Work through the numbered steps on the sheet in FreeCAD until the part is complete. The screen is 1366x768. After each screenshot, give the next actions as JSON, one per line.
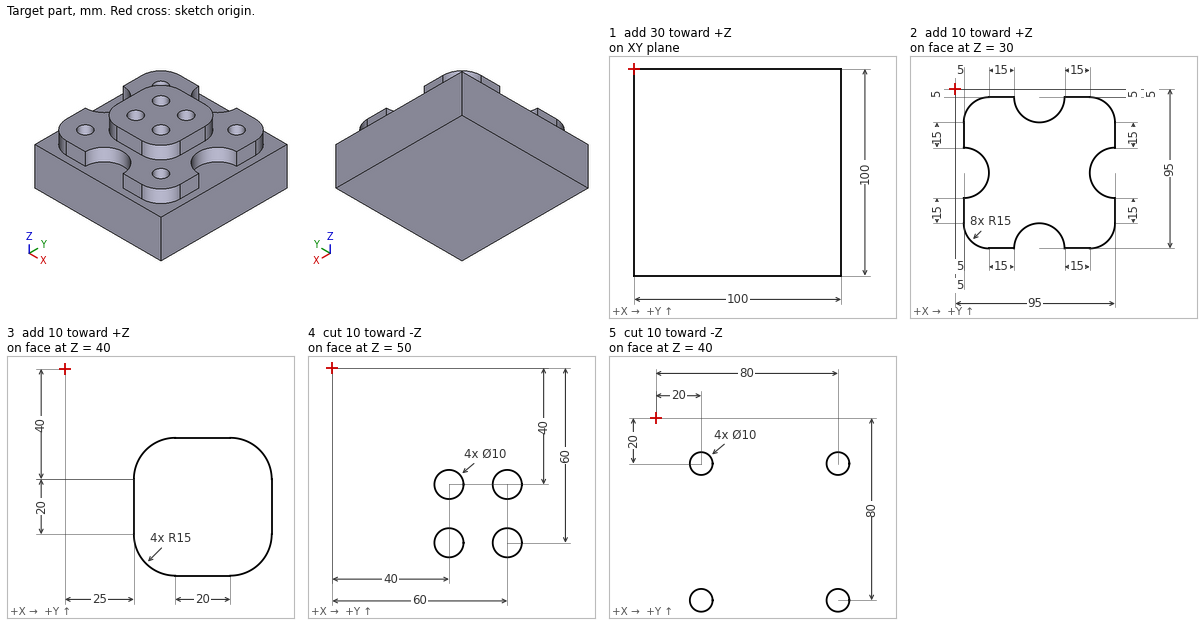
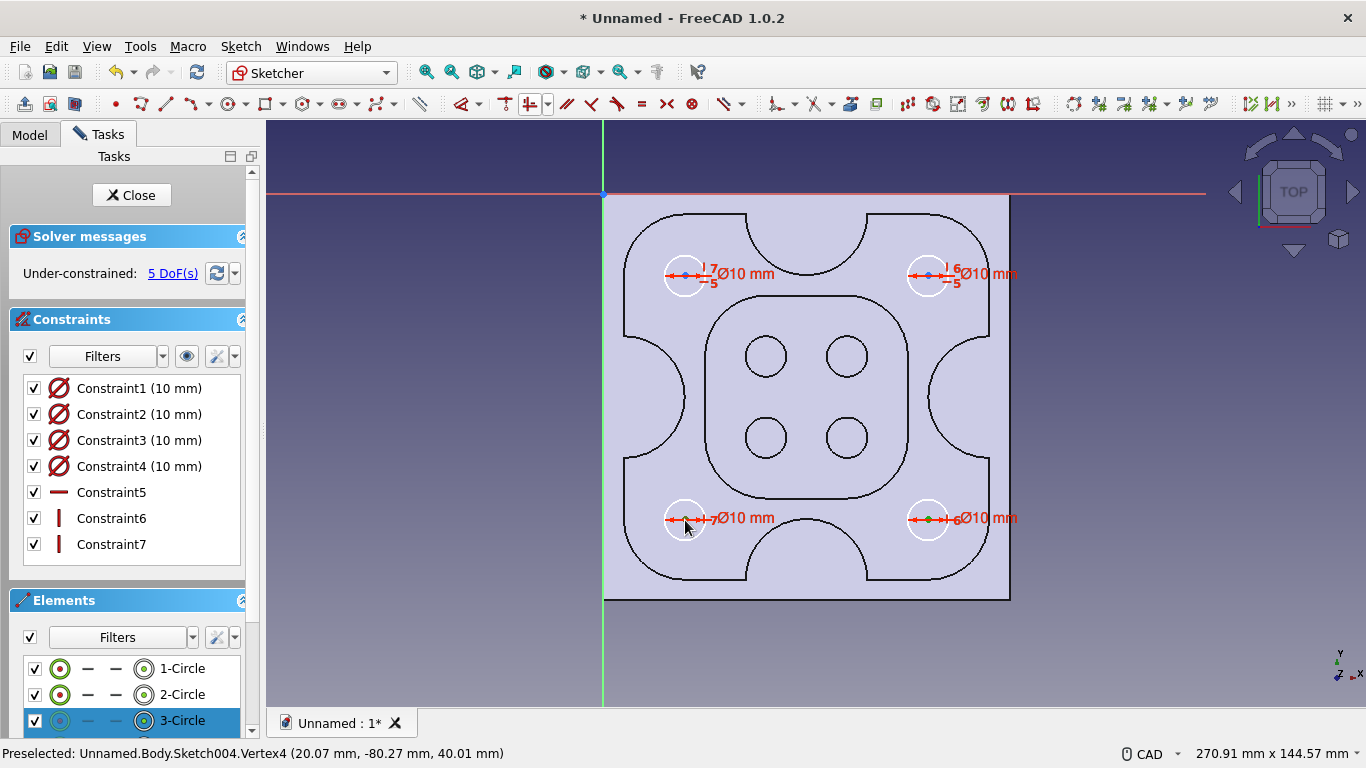
{"action": "left_click", "coordinate": [548, 104]}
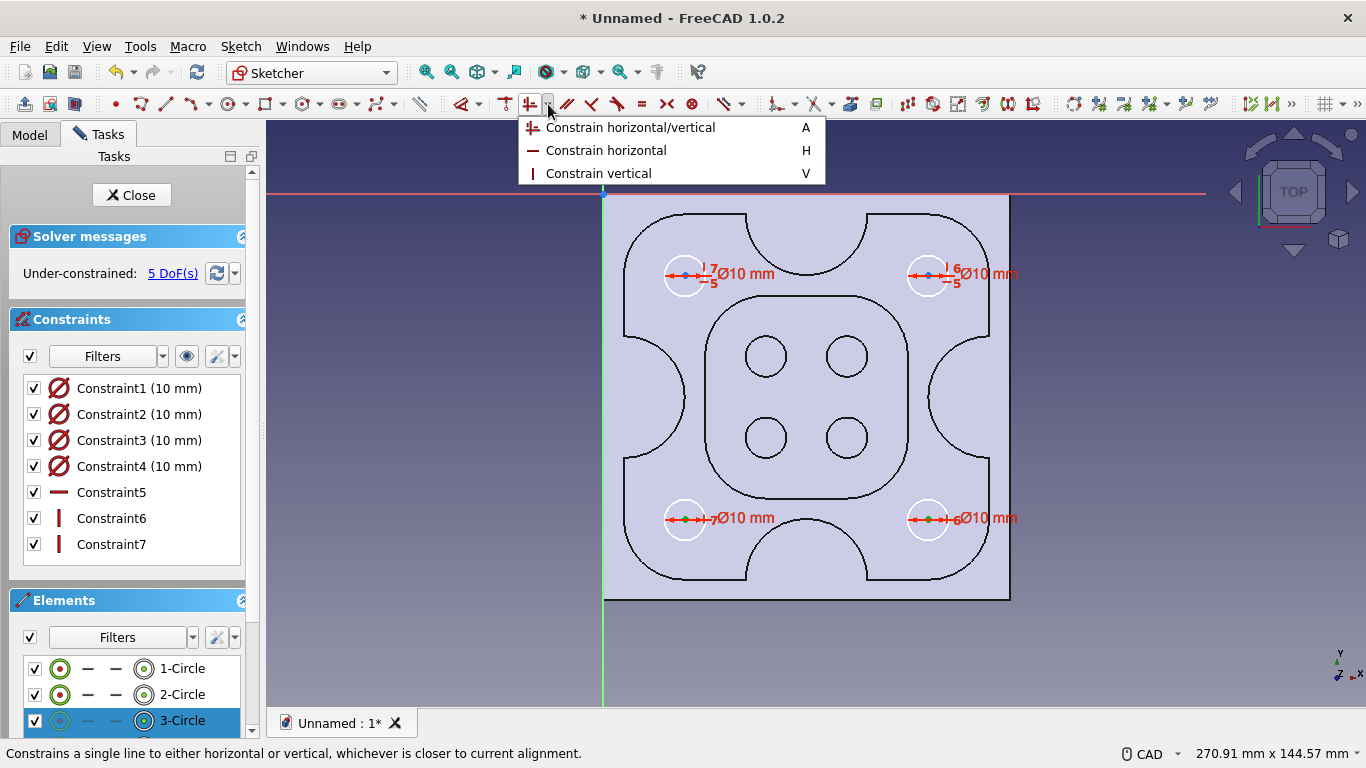
{"action": "left_click", "coordinate": [672, 150]}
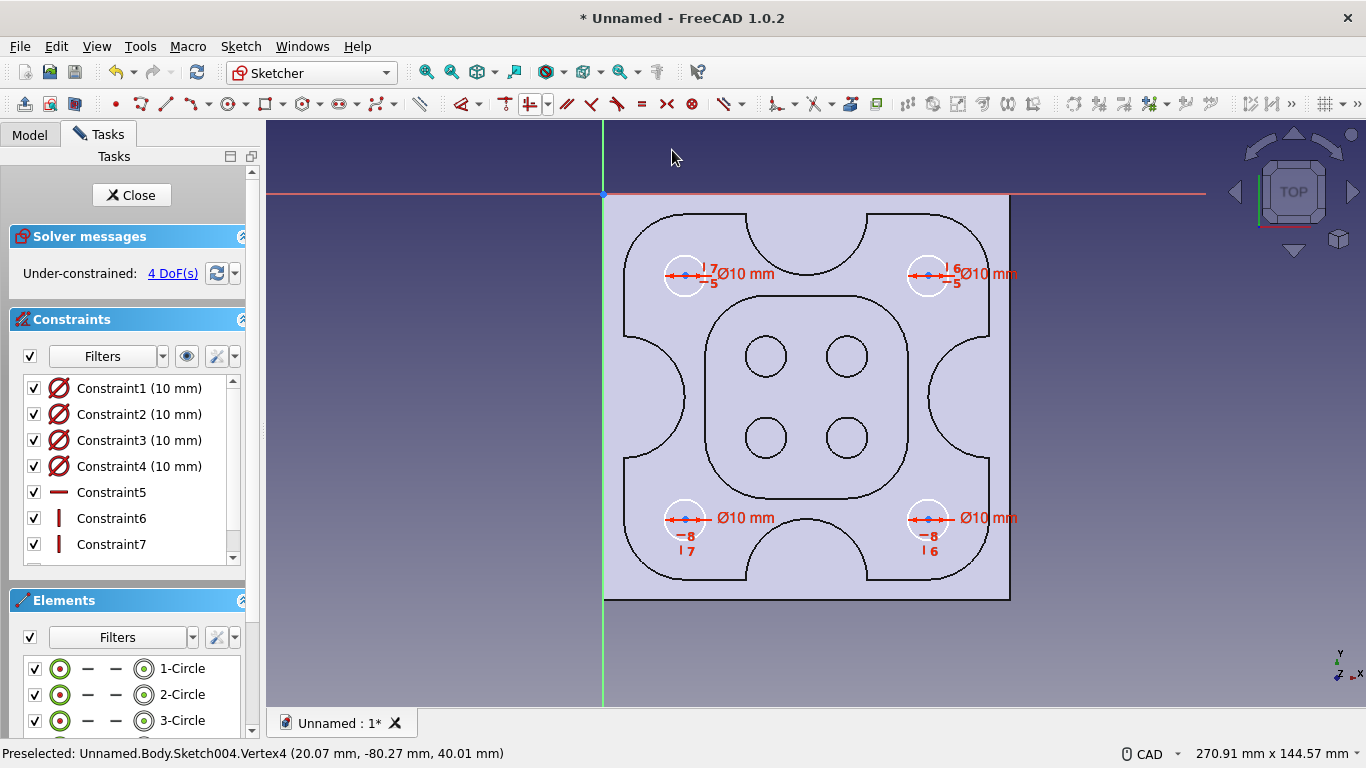
{"action": "left_click", "coordinate": [460, 104]}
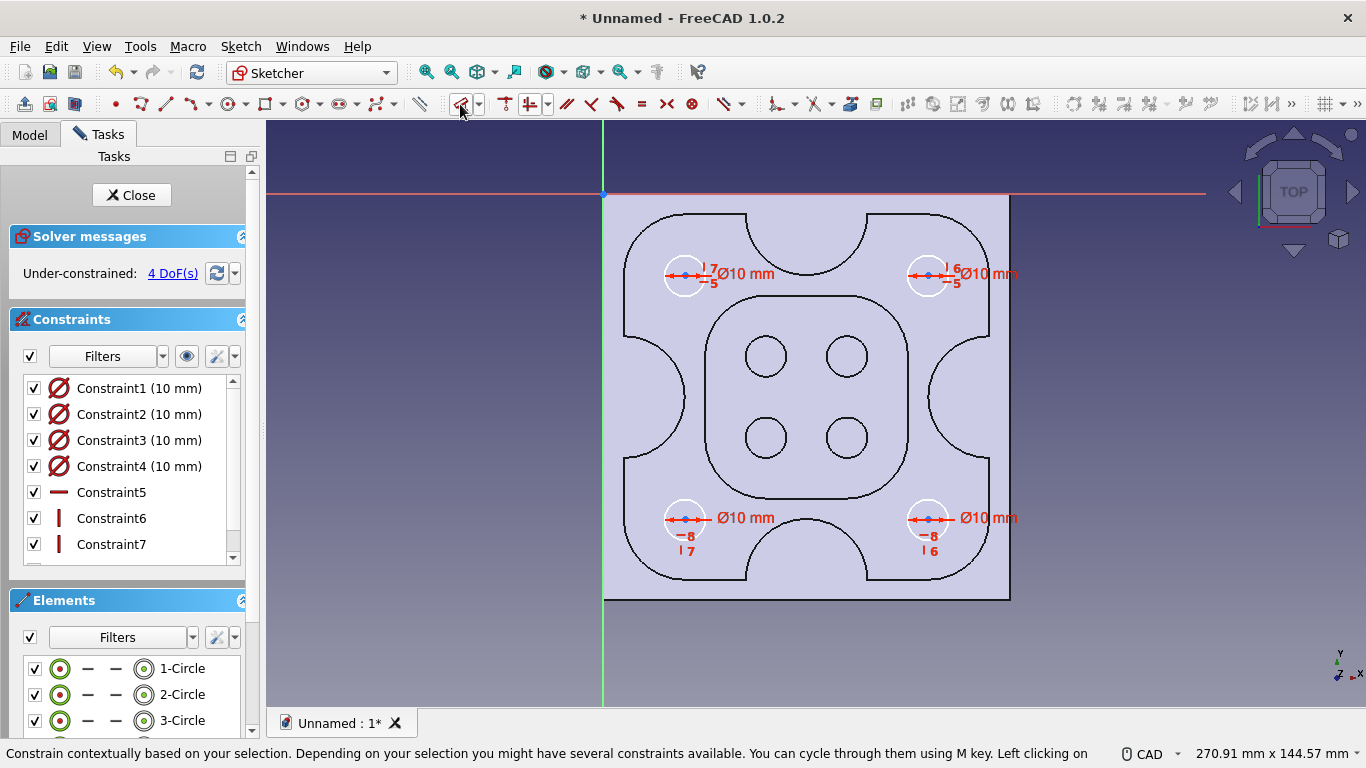
{"action": "left_click", "coordinate": [685, 276]}
{"action": "left_click", "coordinate": [644, 160]}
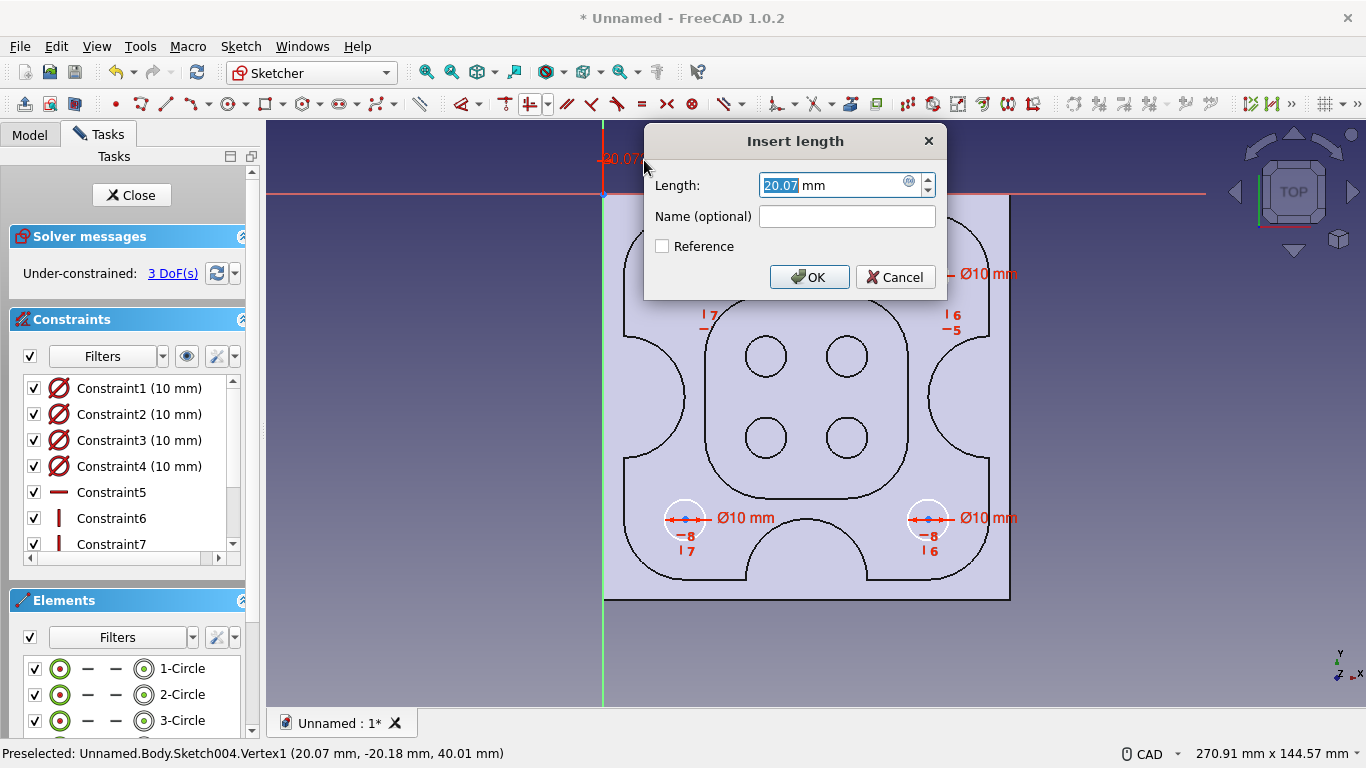
{"action": "type", "text": "20"}
{"action": "key", "text": "Return"}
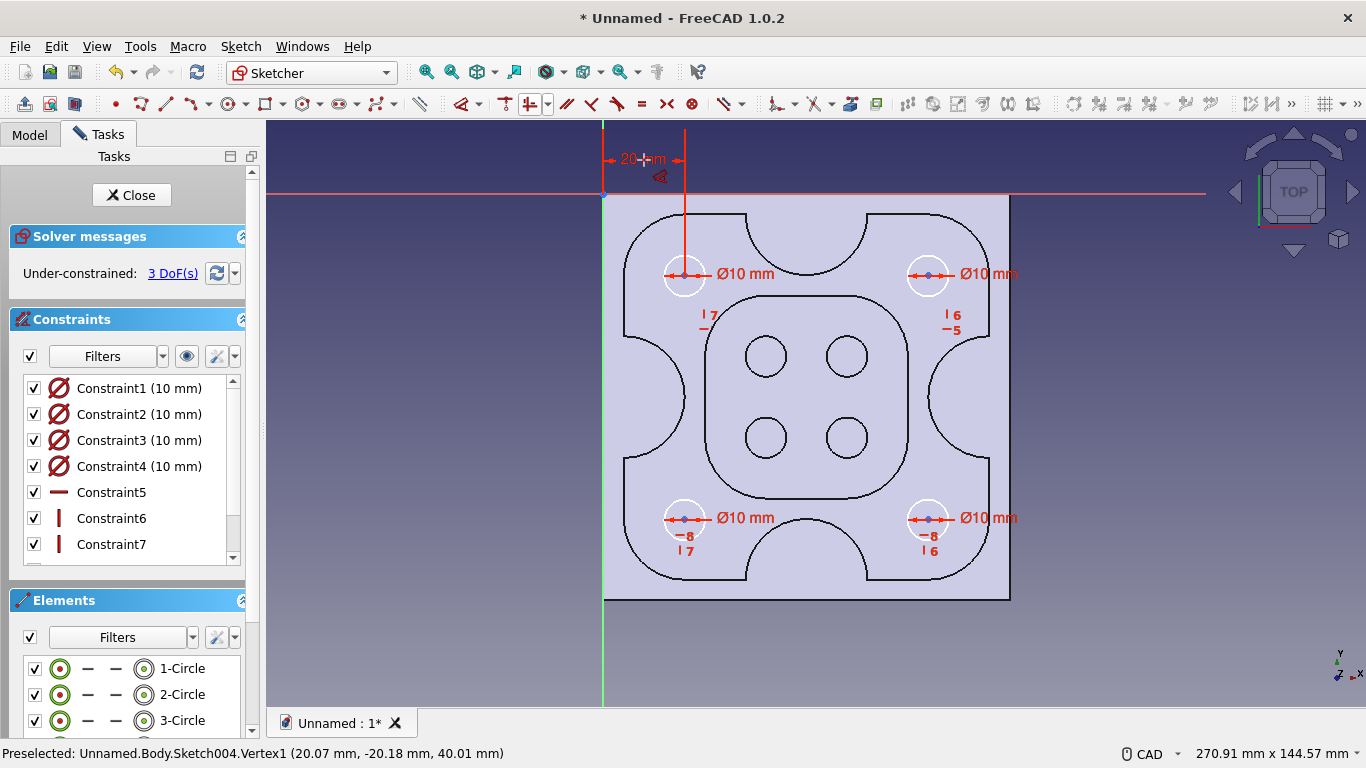
{"action": "left_click", "coordinate": [685, 276]}
{"action": "left_click", "coordinate": [569, 235]}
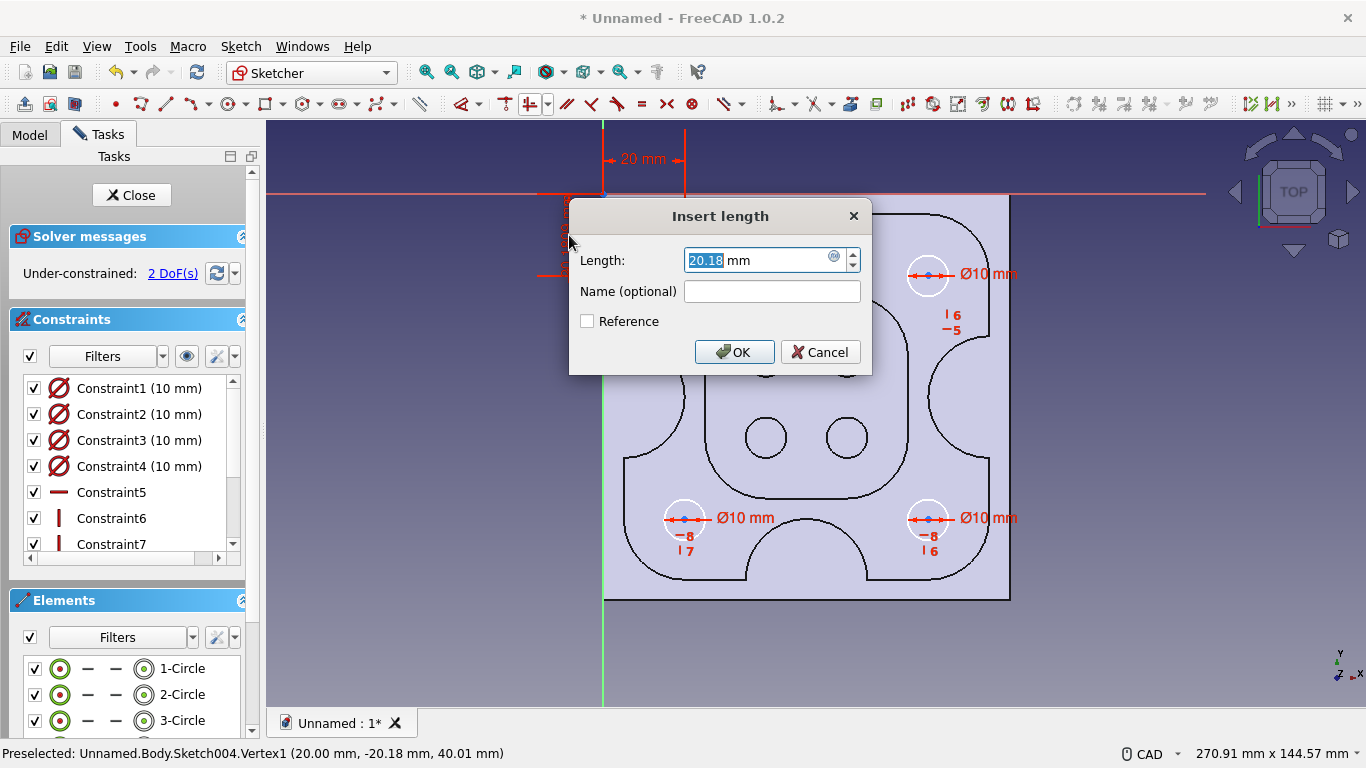
{"action": "type", "text": "20"}
{"action": "key", "text": "Return"}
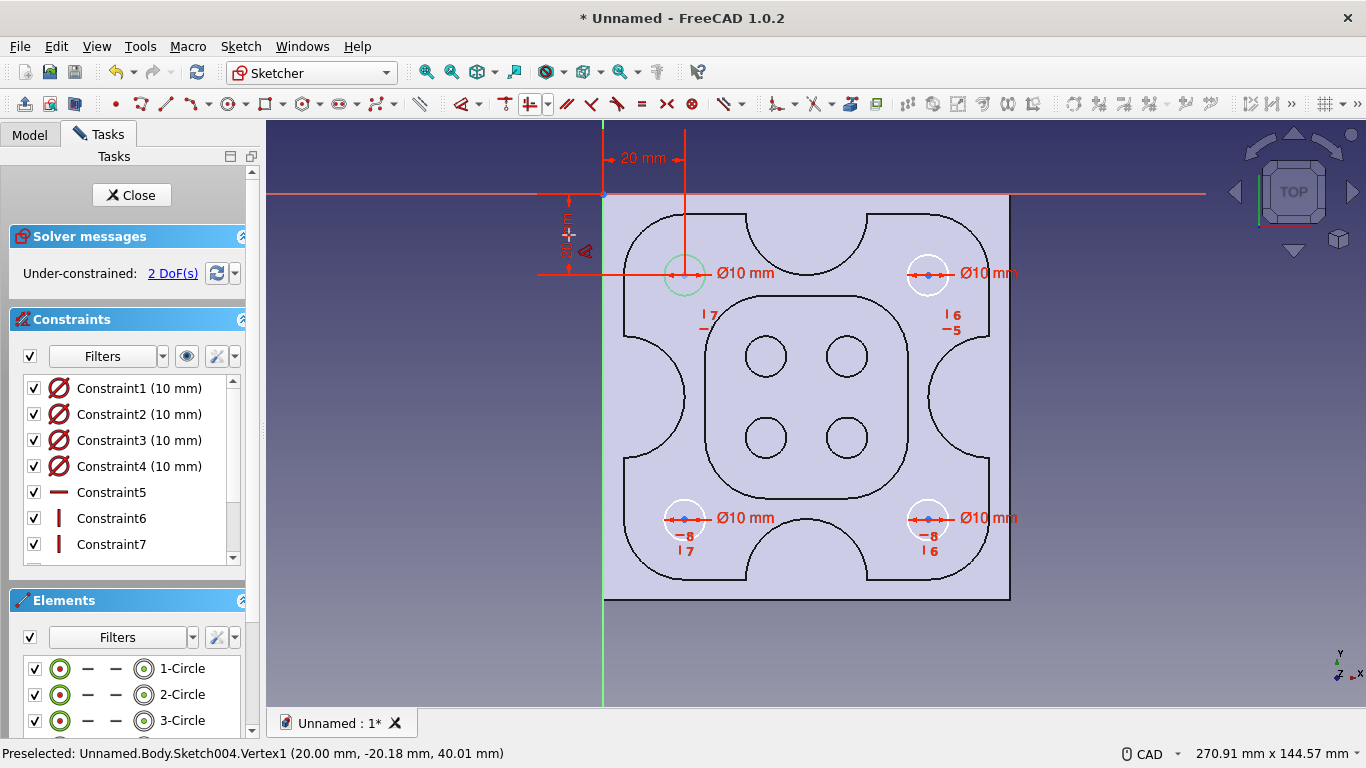
{"action": "left_click", "coordinate": [928, 275]}
{"action": "left_click", "coordinate": [766, 160]}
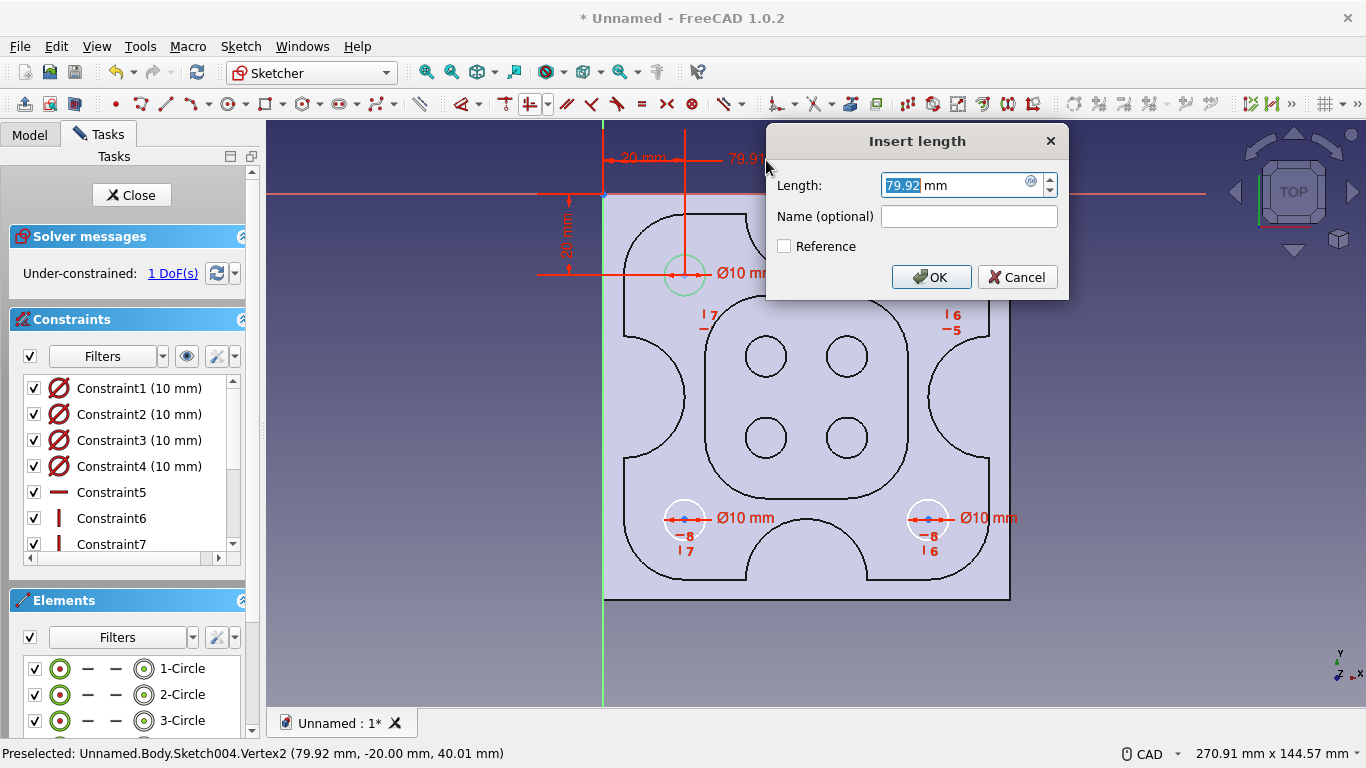
{"action": "type", "text": "80"}
{"action": "key", "text": "Return"}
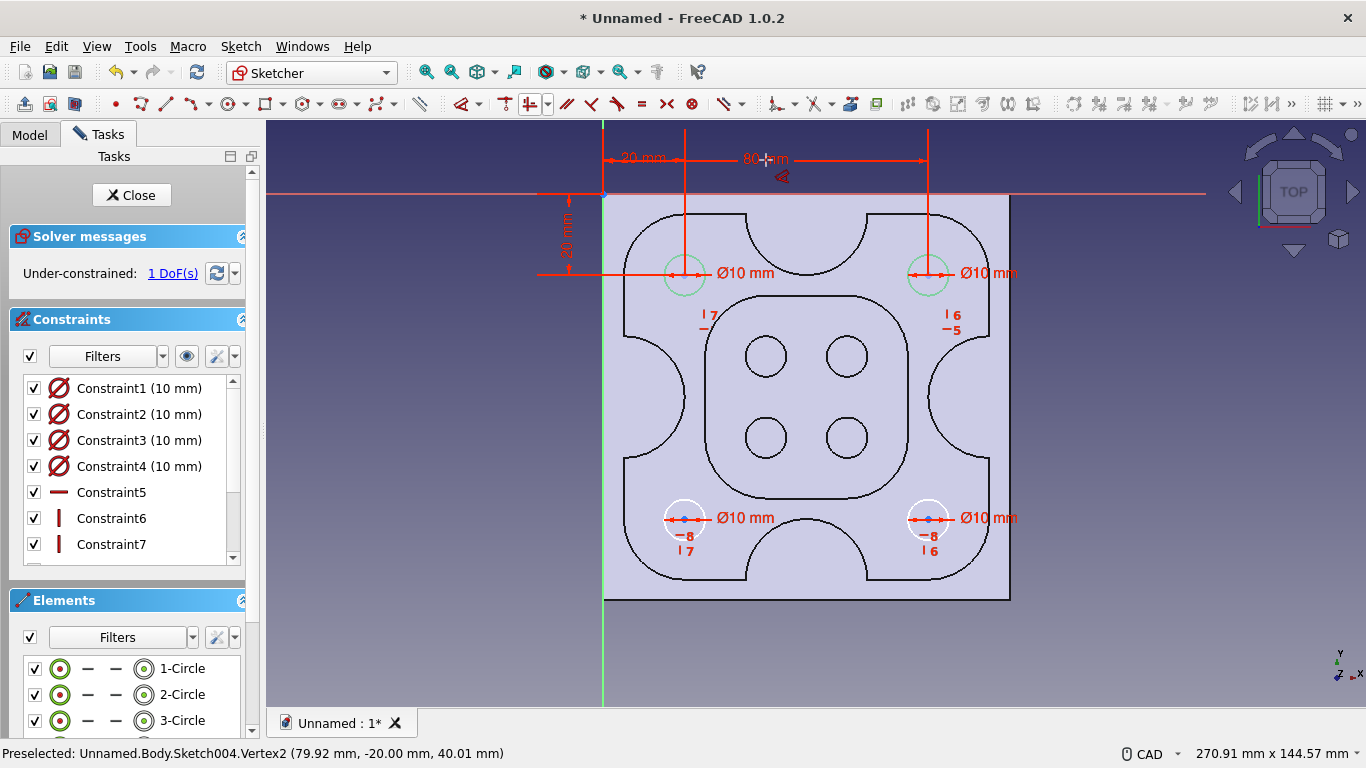
{"action": "left_click", "coordinate": [928, 520]}
{"action": "left_click", "coordinate": [569, 357]}